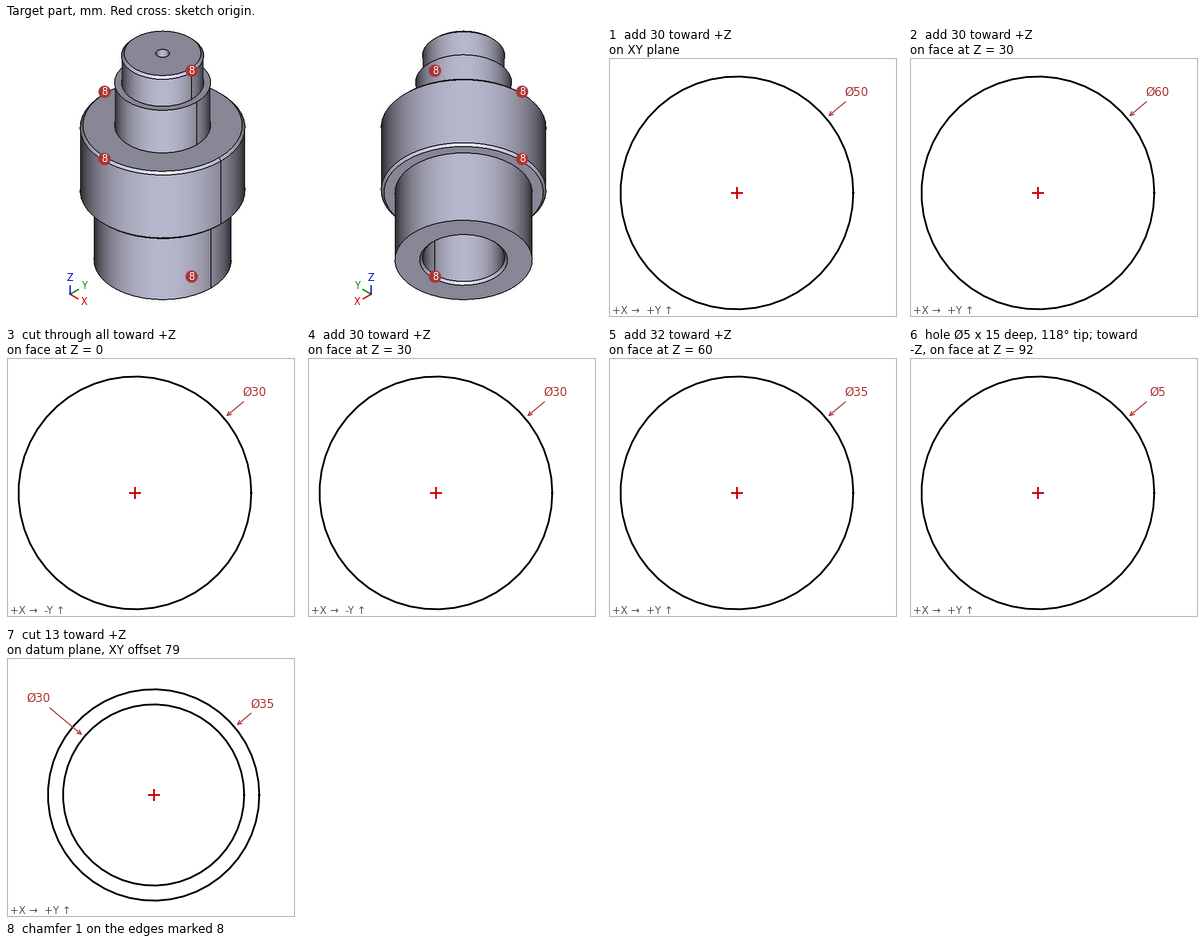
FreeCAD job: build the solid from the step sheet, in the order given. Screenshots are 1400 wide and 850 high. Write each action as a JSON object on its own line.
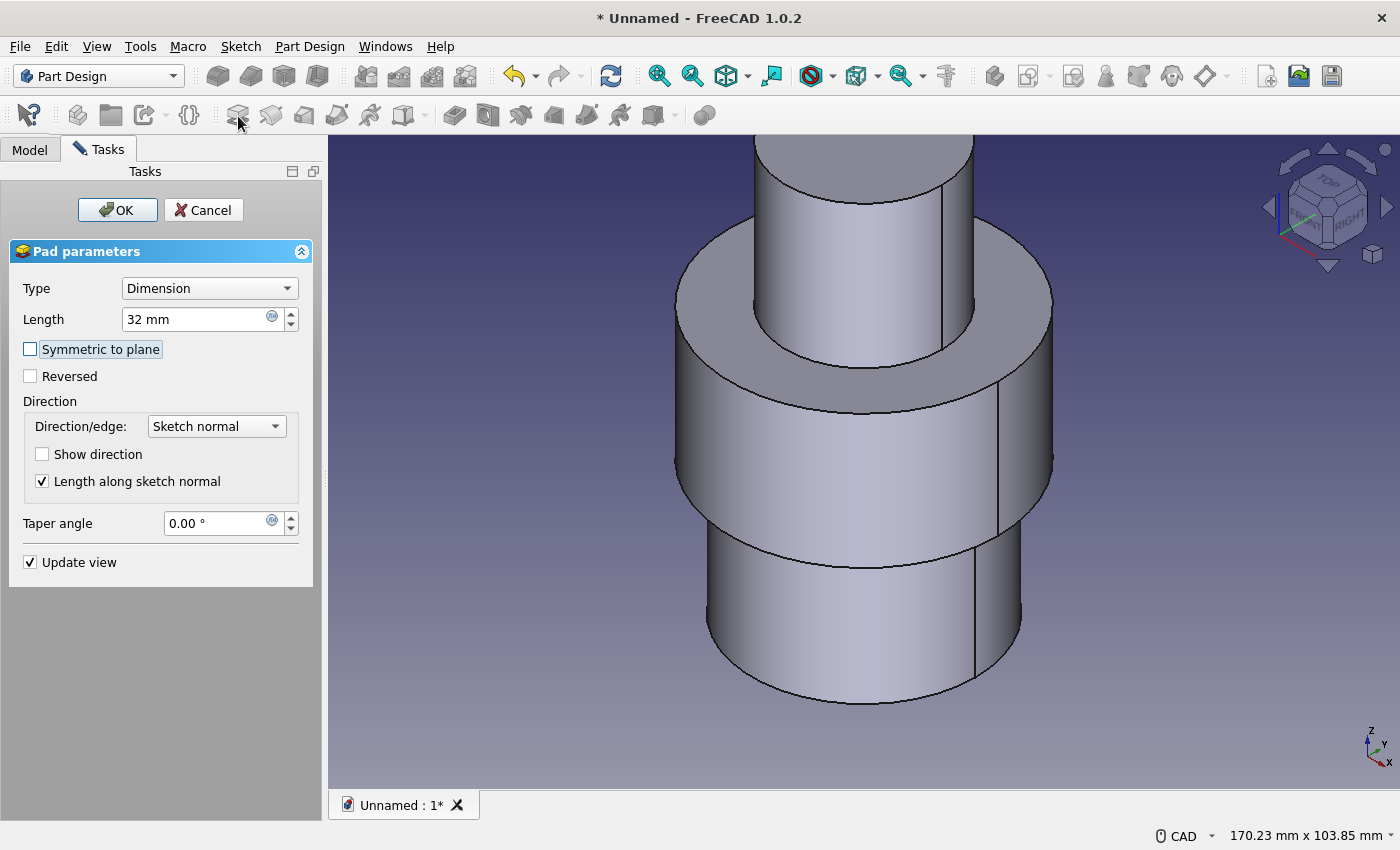
{"action": "left_click", "coordinate": [118, 210]}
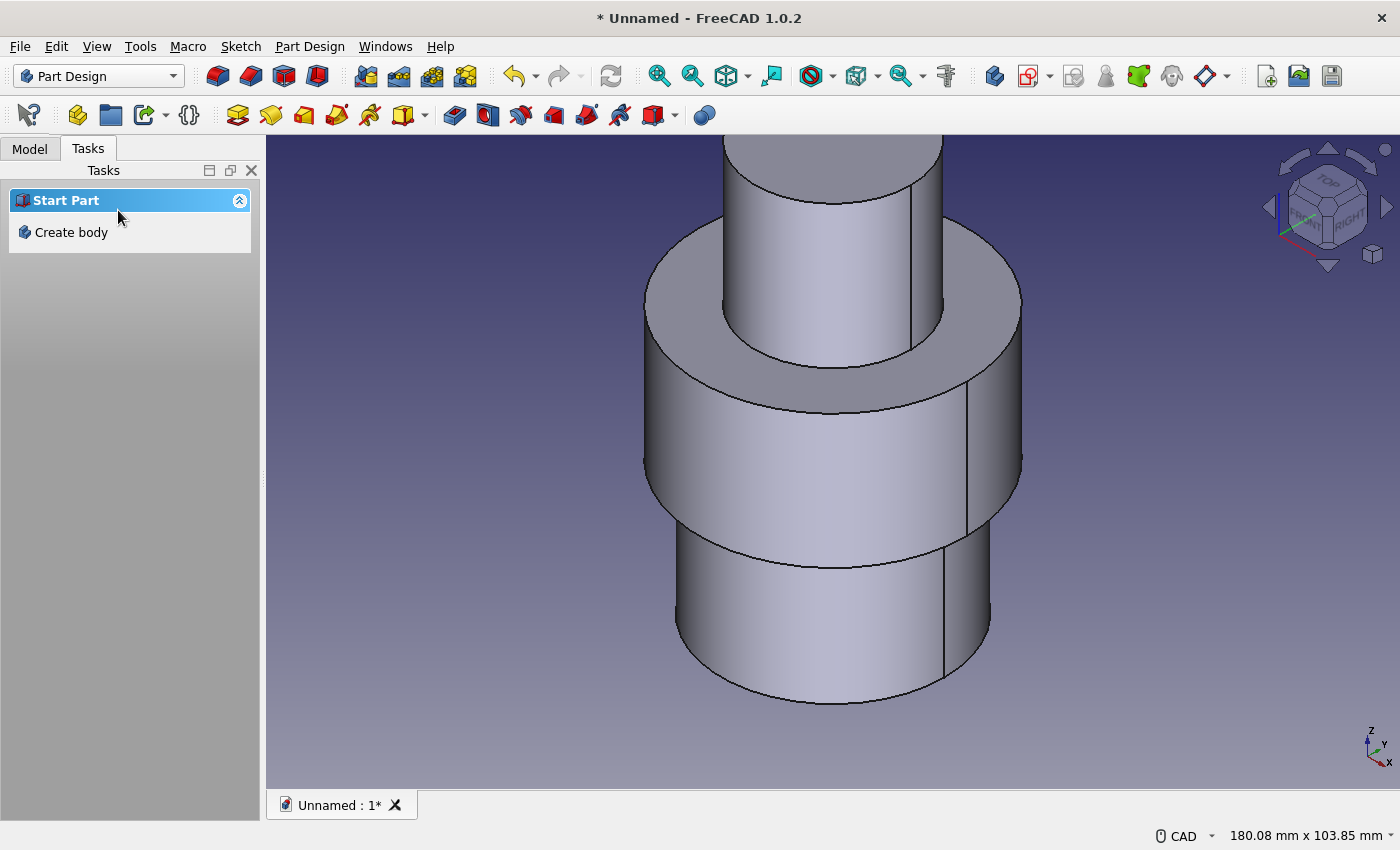
{"action": "key", "text": "v f"}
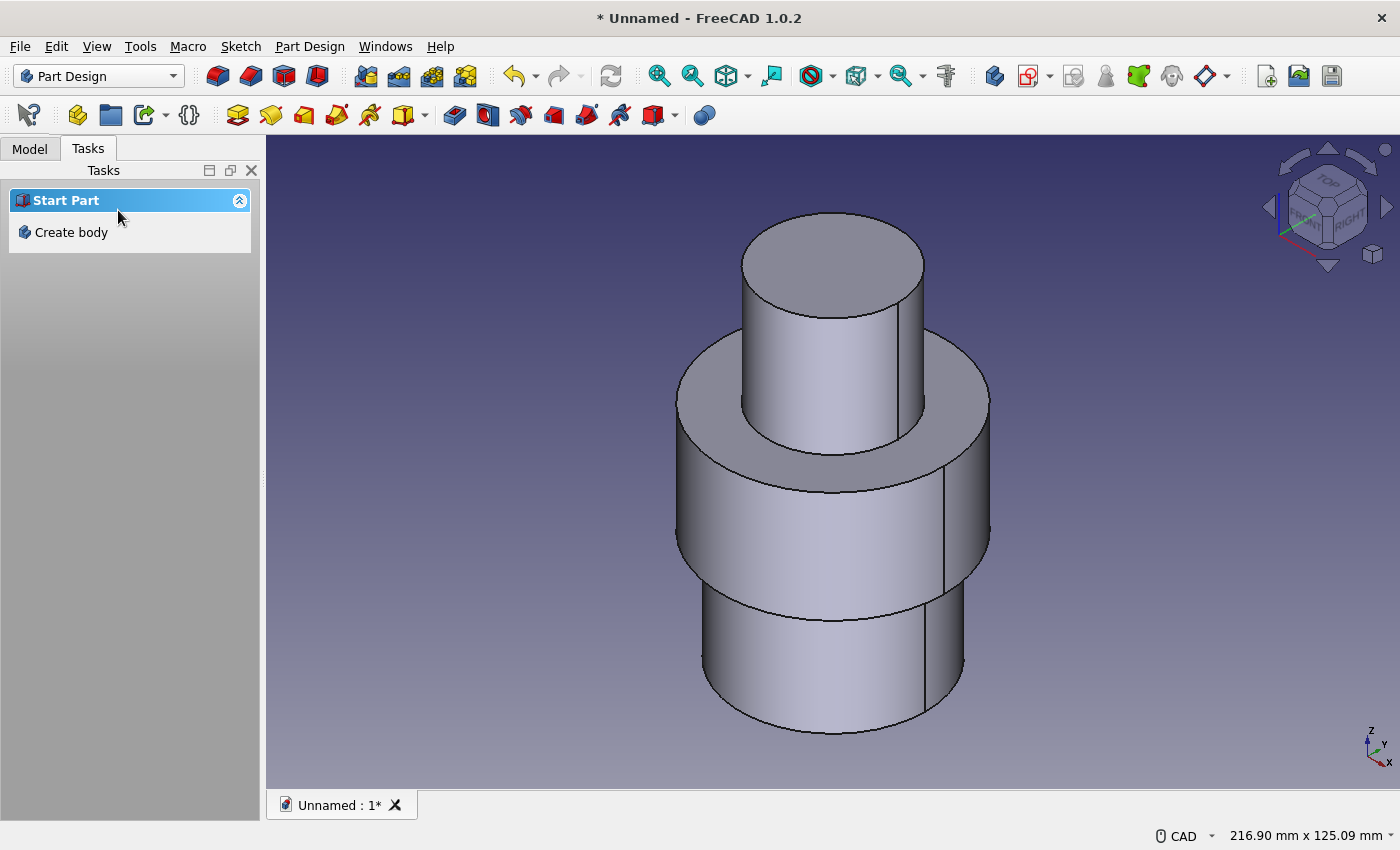
{"action": "left_click", "coordinate": [833, 265]}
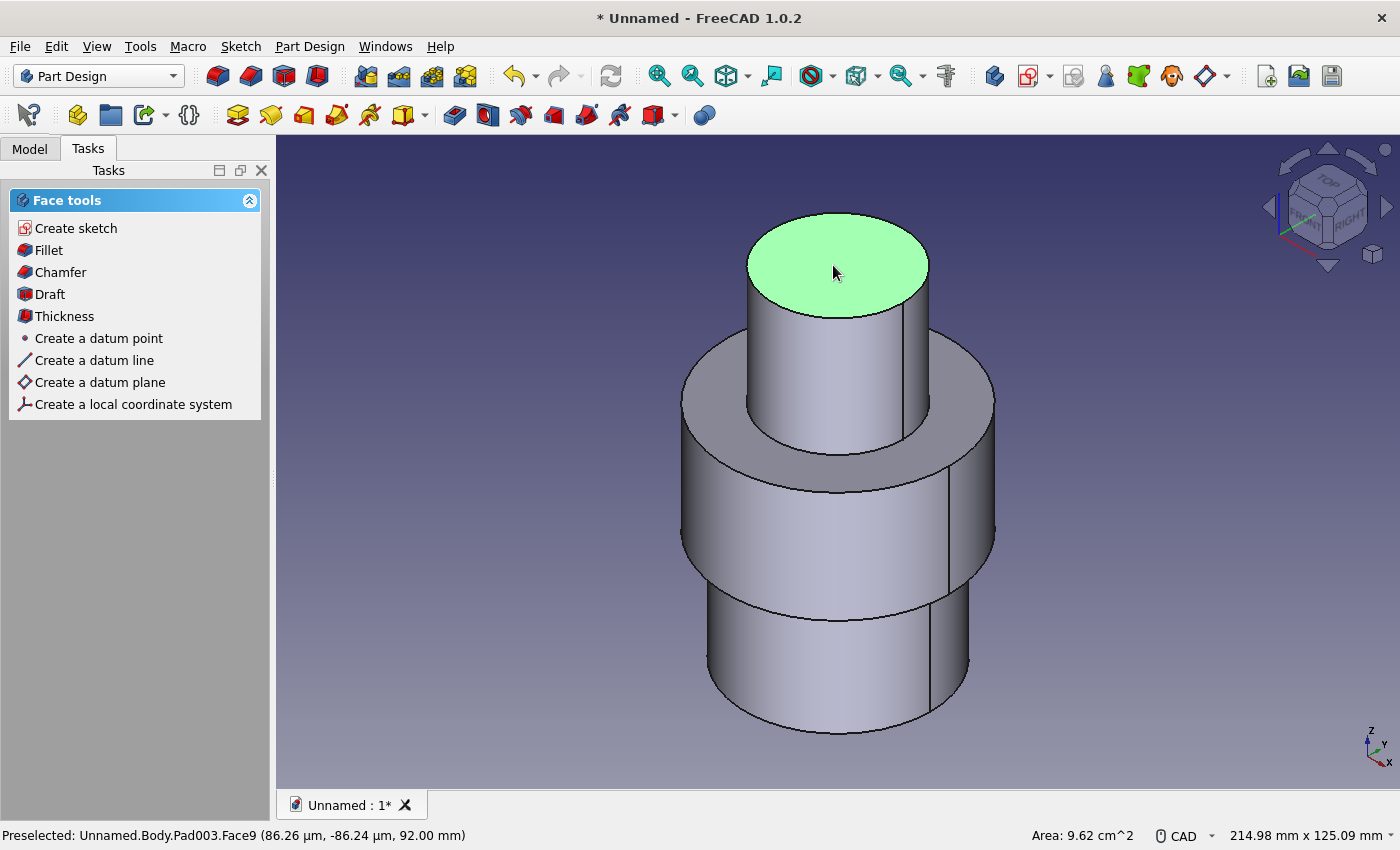
{"action": "left_click", "coordinate": [1028, 76]}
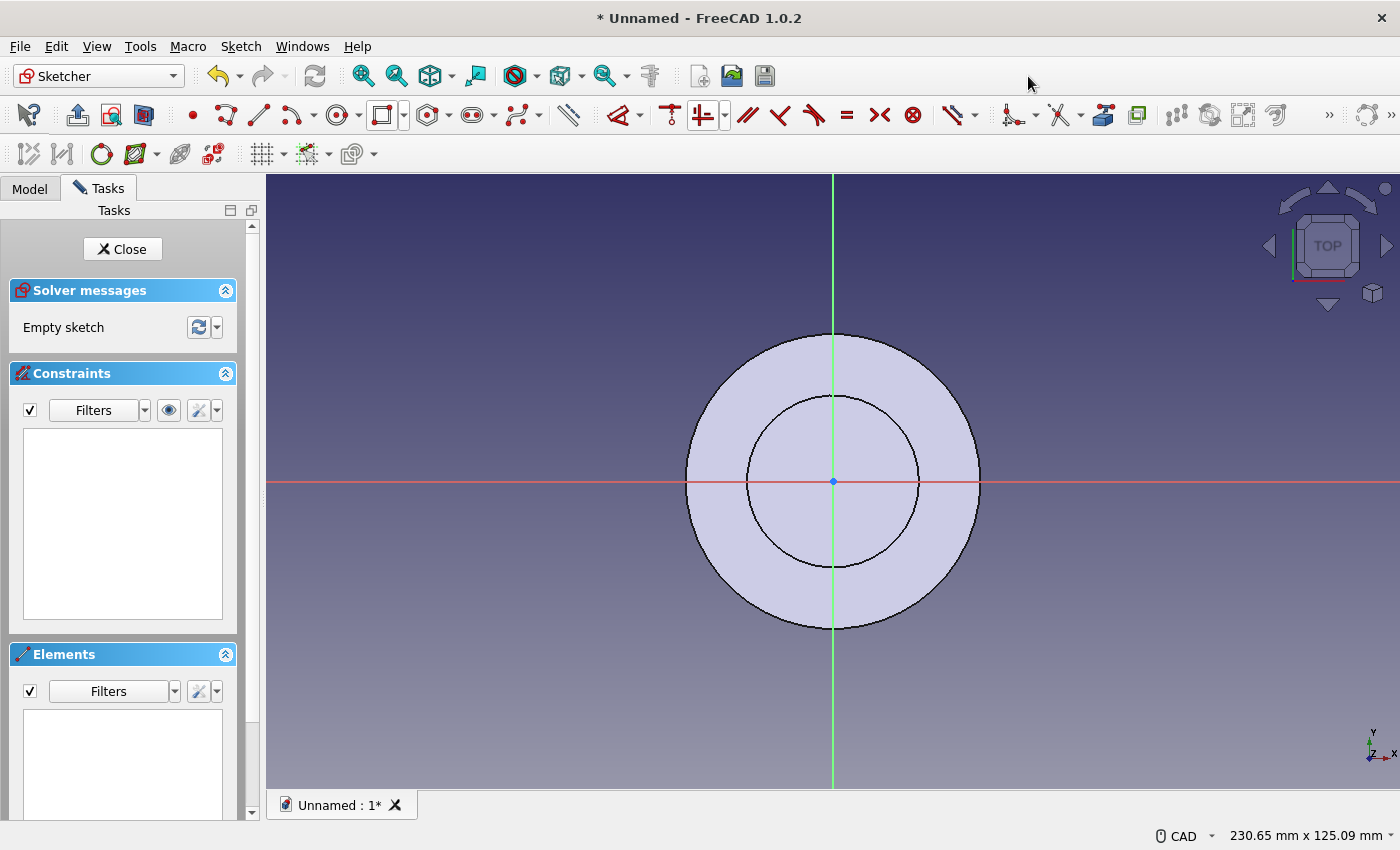
{"action": "scroll", "coordinate": [837, 482], "scroll_direction": "up", "scroll_amount": 14}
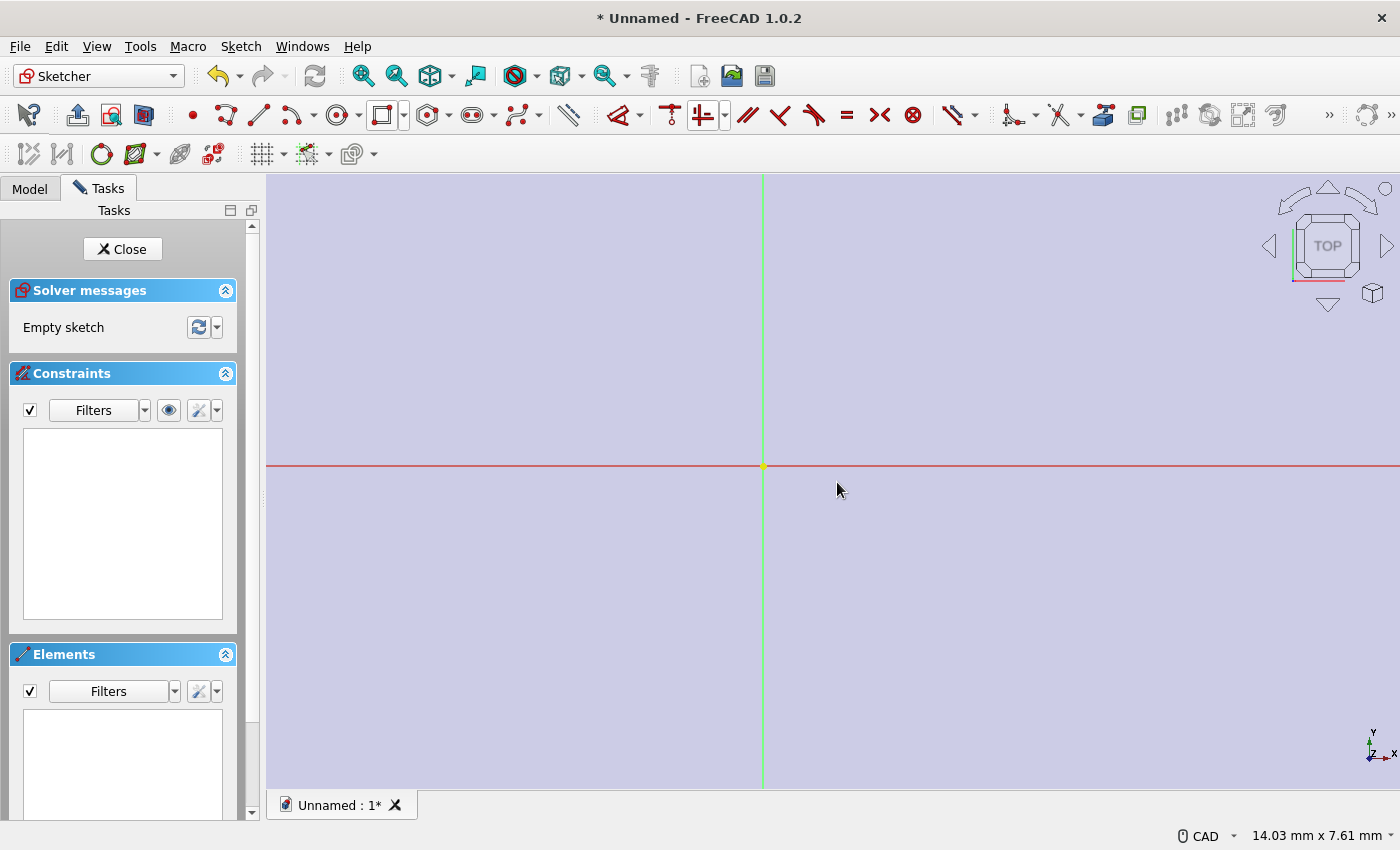
{"action": "key", "text": "g c"}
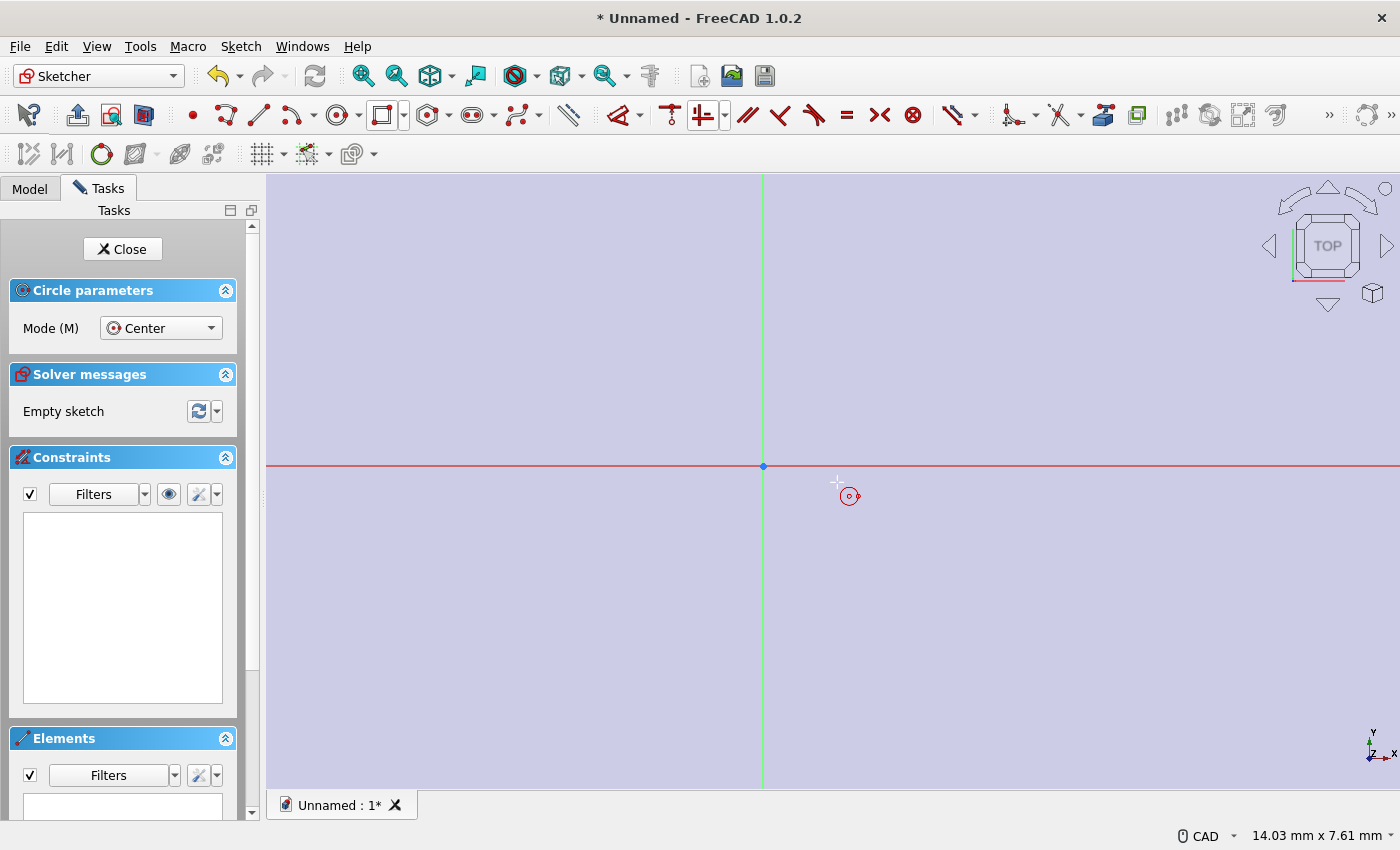
{"action": "left_click", "coordinate": [763, 466]}
{"action": "left_click", "coordinate": [906, 323]}
{"action": "key", "text": "Escape"}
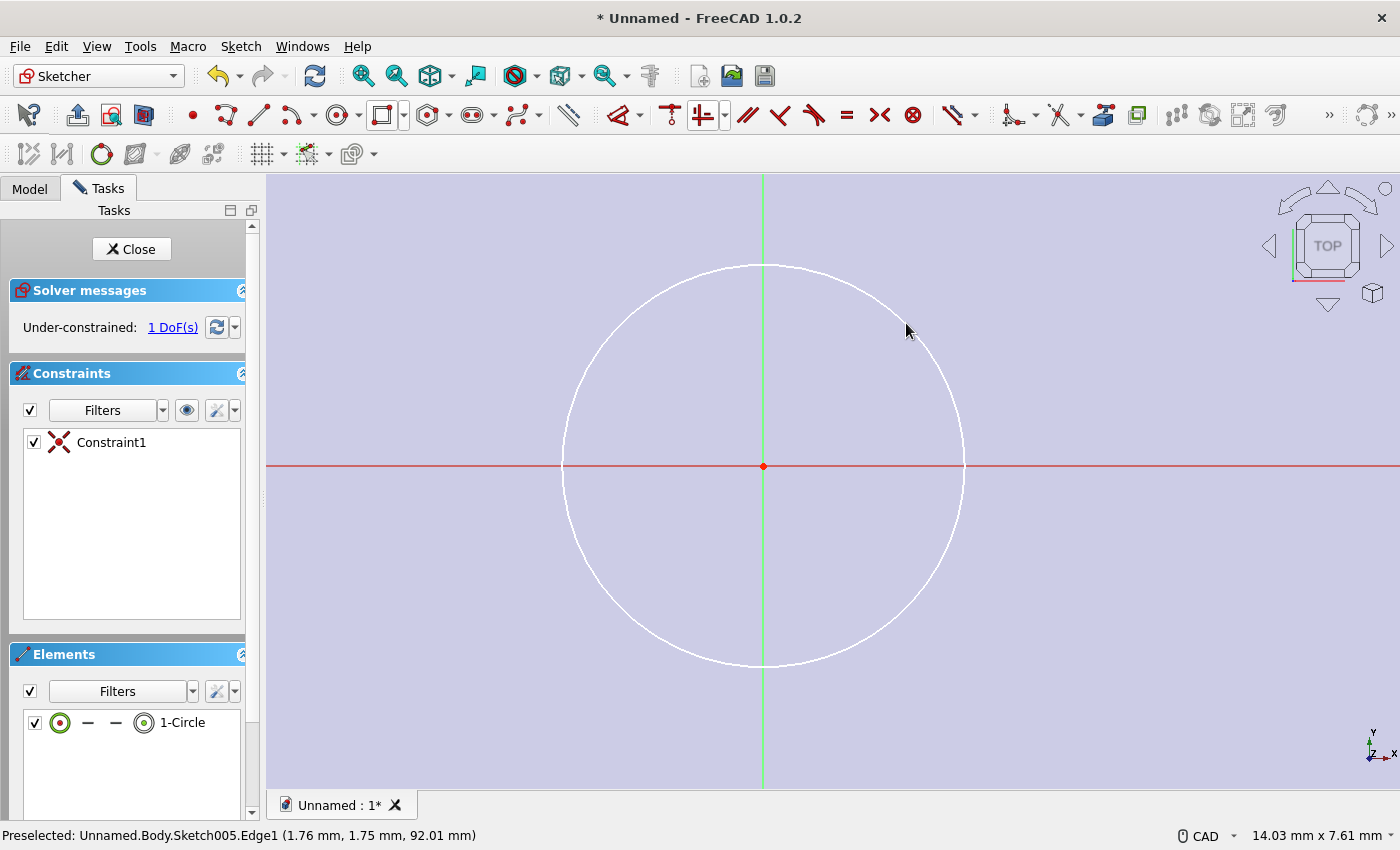
{"action": "key", "text": "d"}